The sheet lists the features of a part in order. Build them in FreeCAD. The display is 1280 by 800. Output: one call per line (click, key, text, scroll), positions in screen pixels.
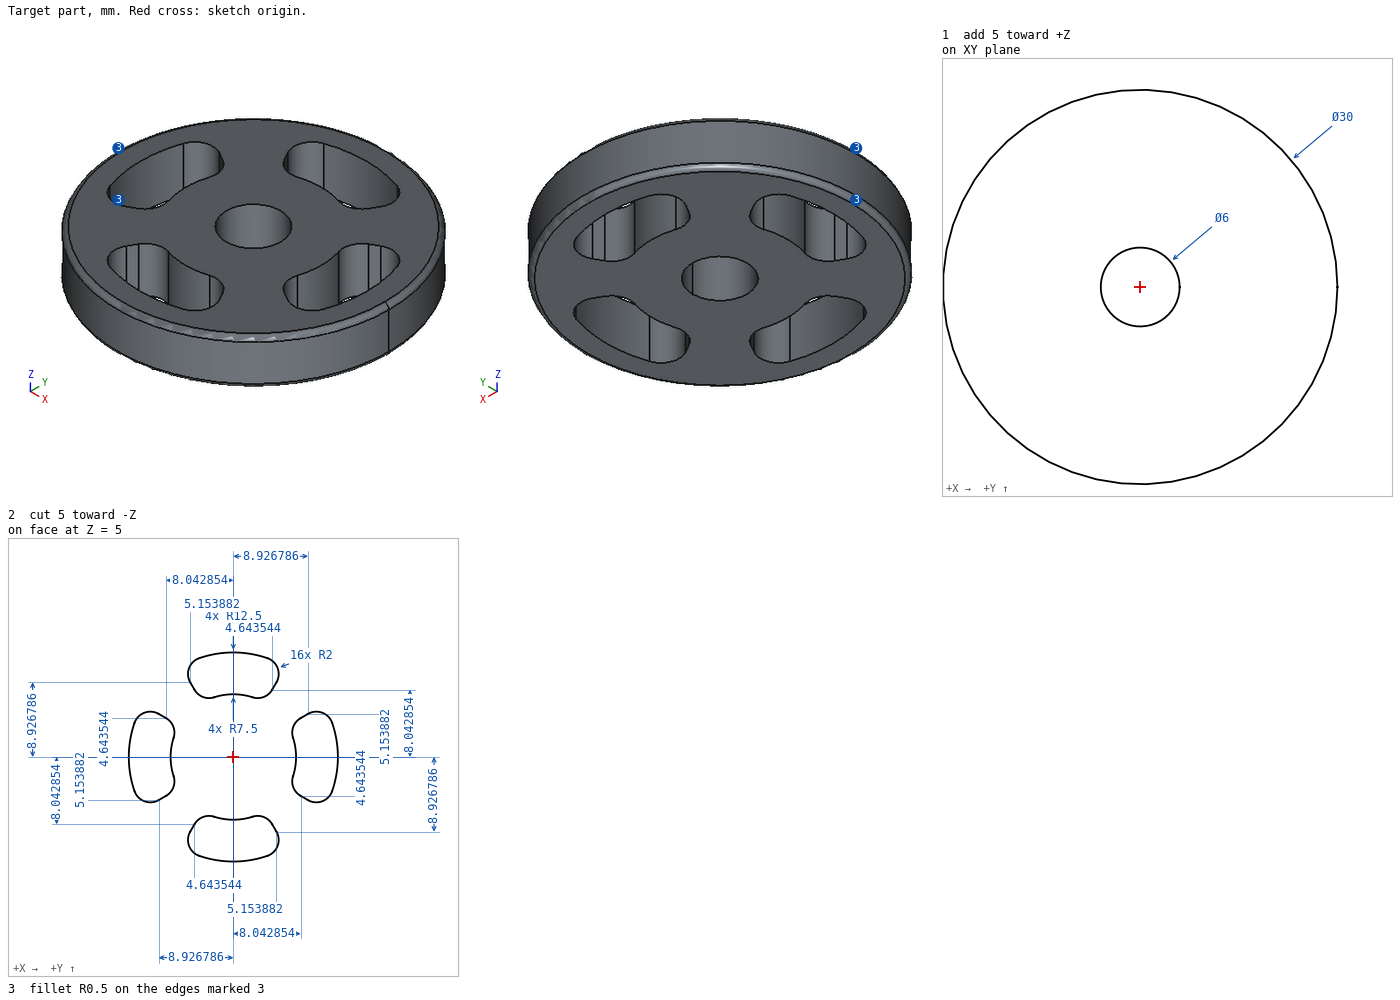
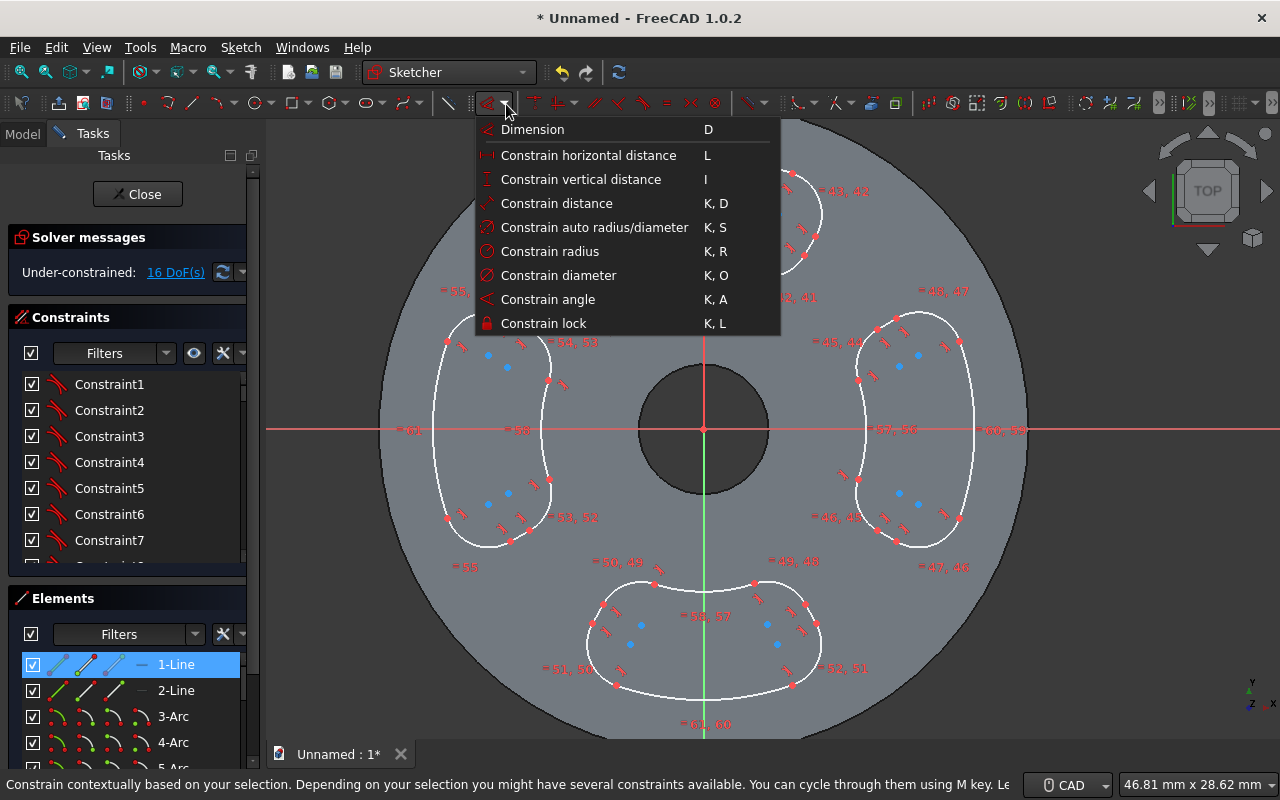
click(628, 155)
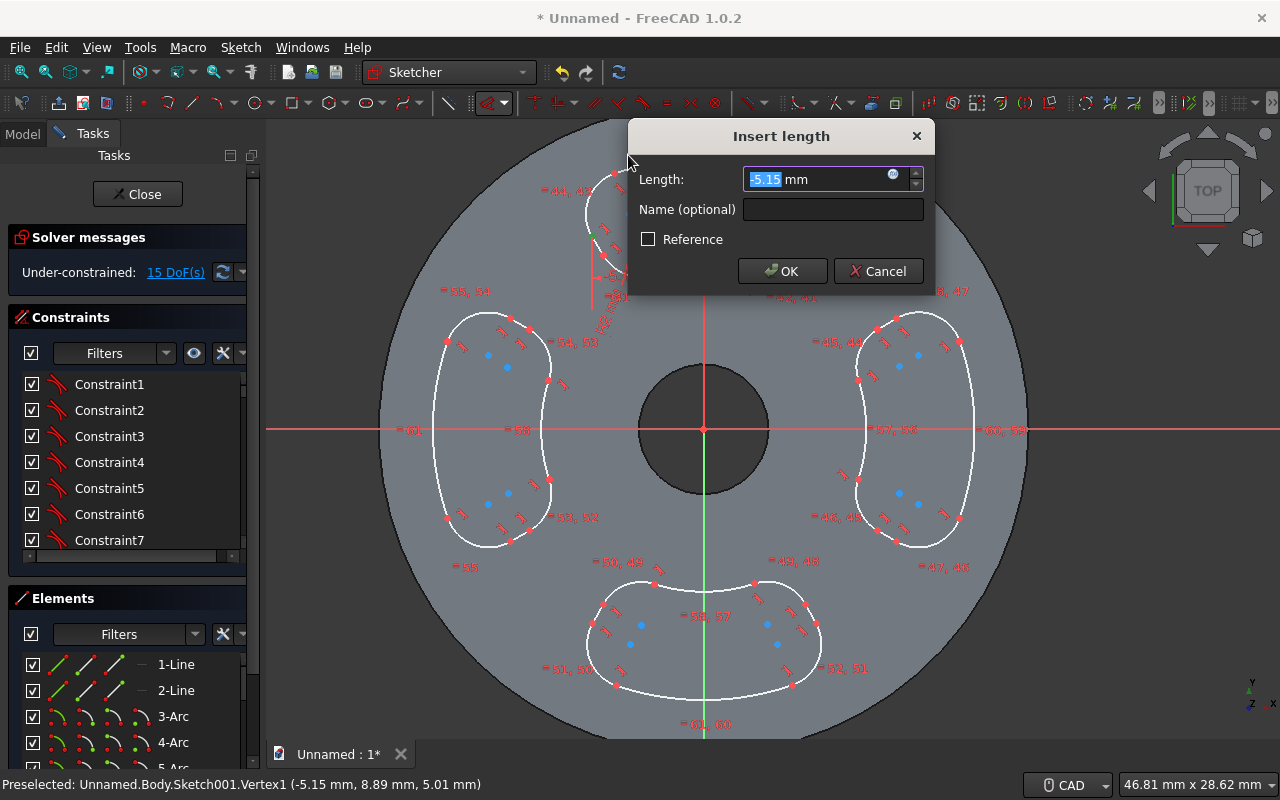
text(-5.153882)
key(Return)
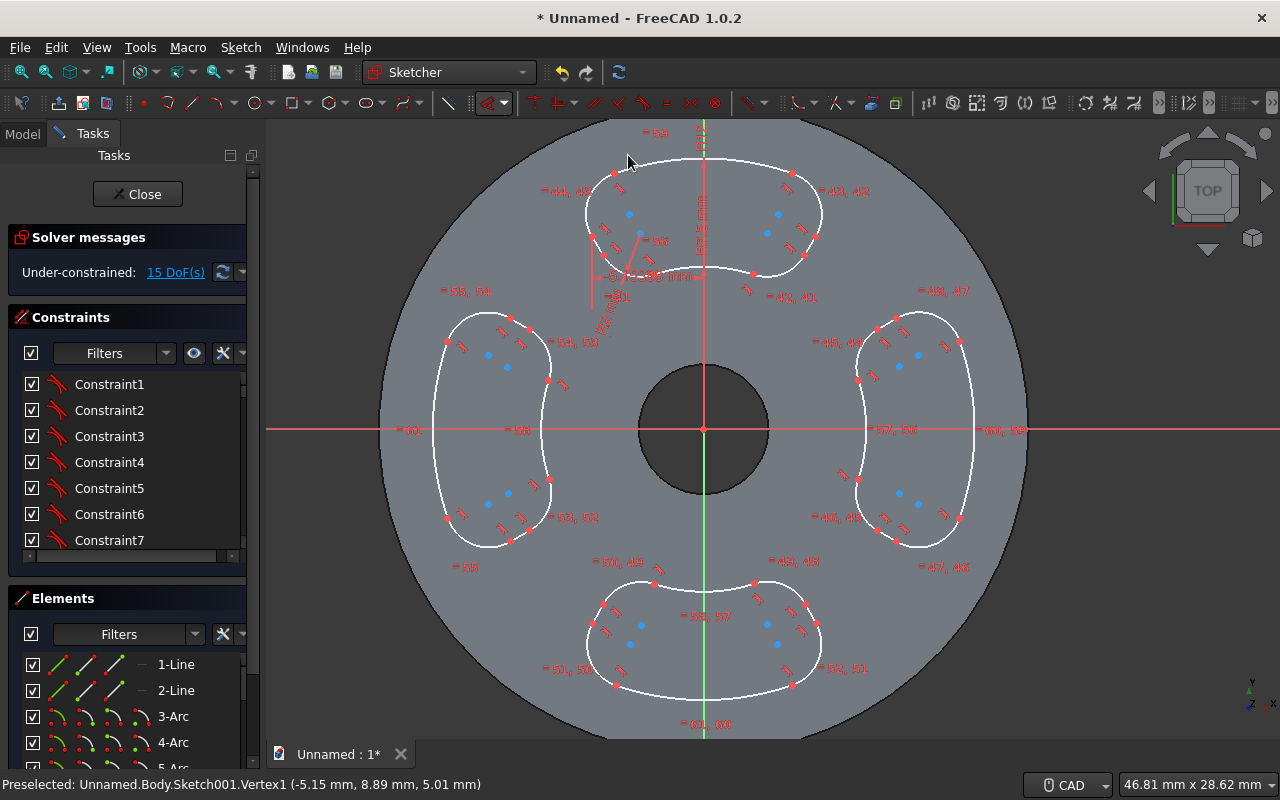
click(592, 237)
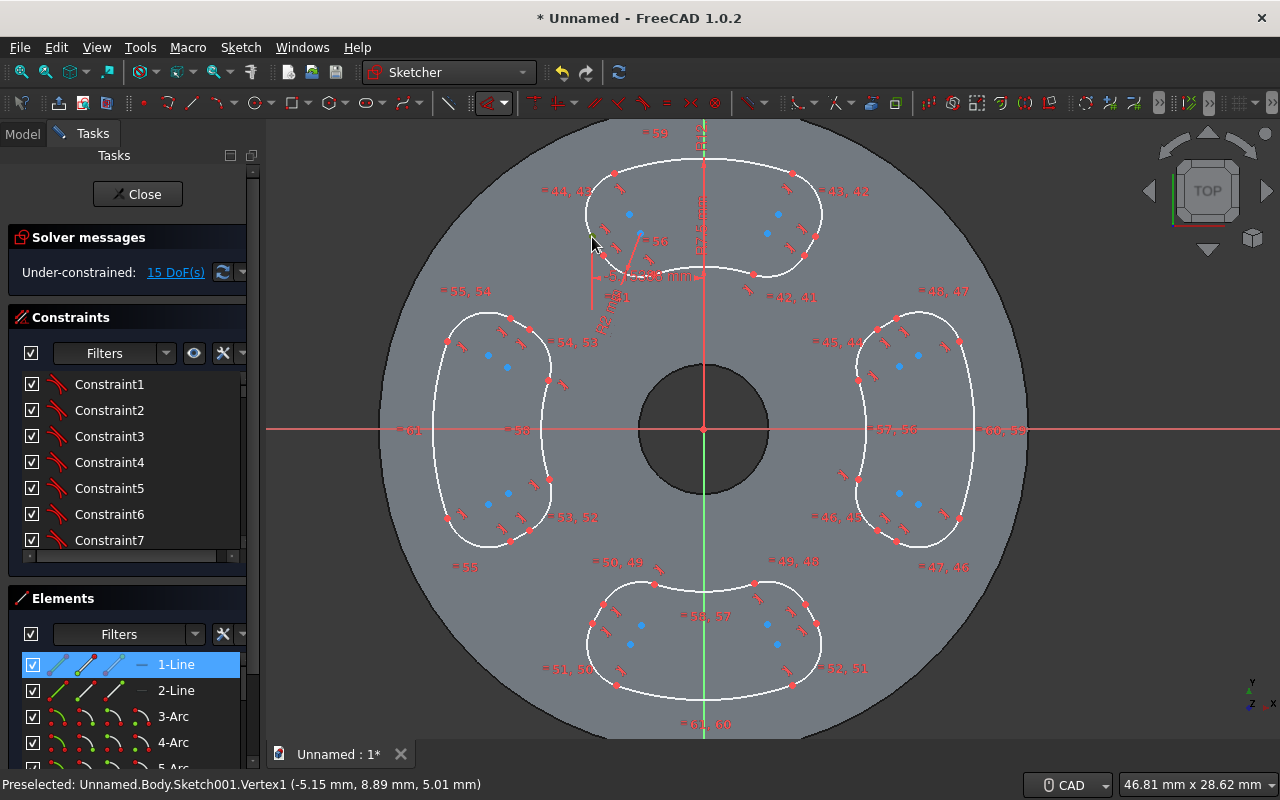
click(506, 104)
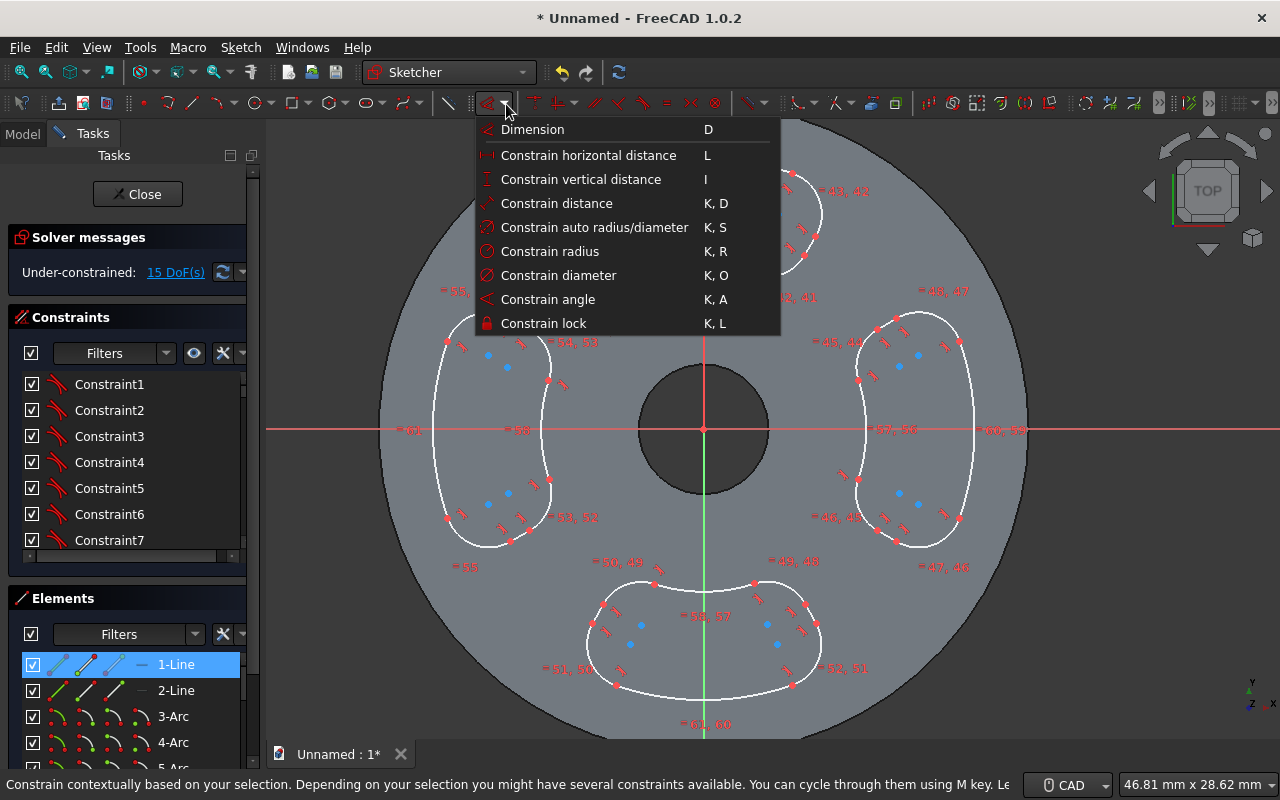
click(628, 179)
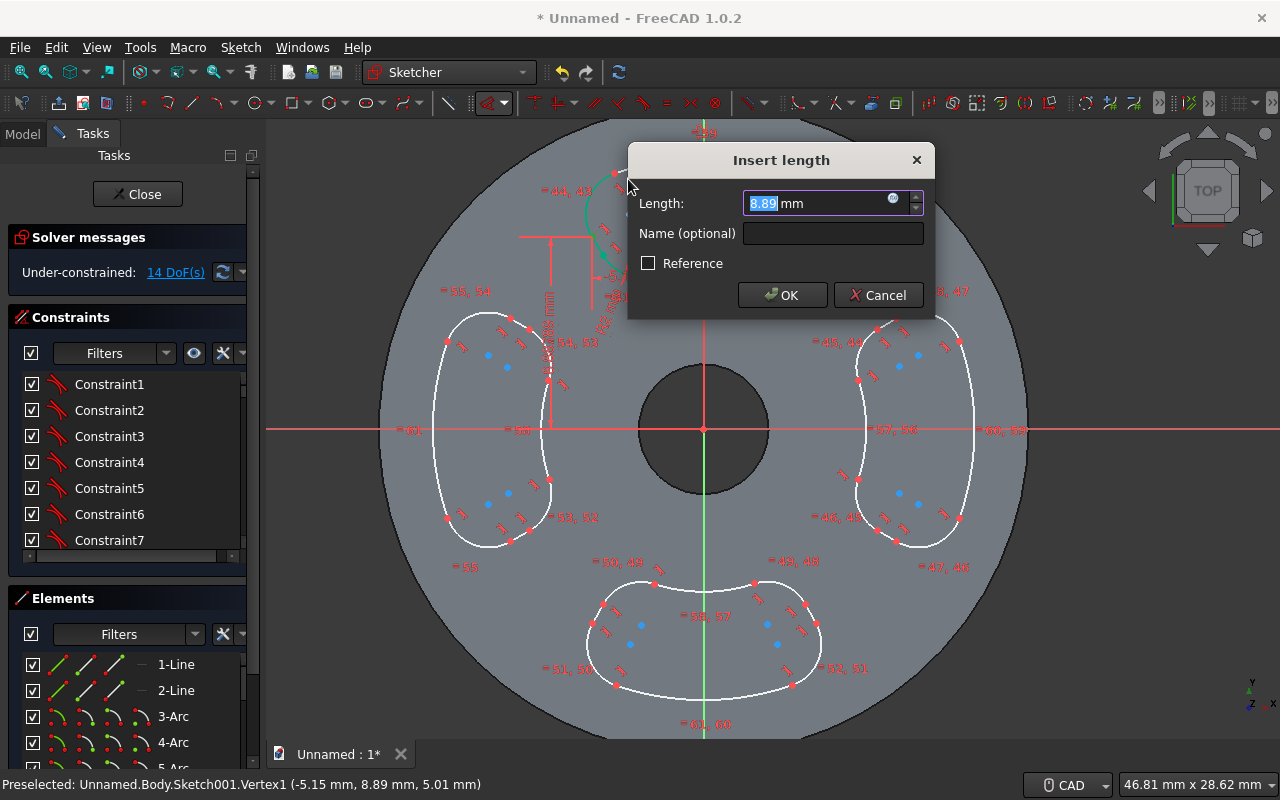
text(8.926786)
key(Return)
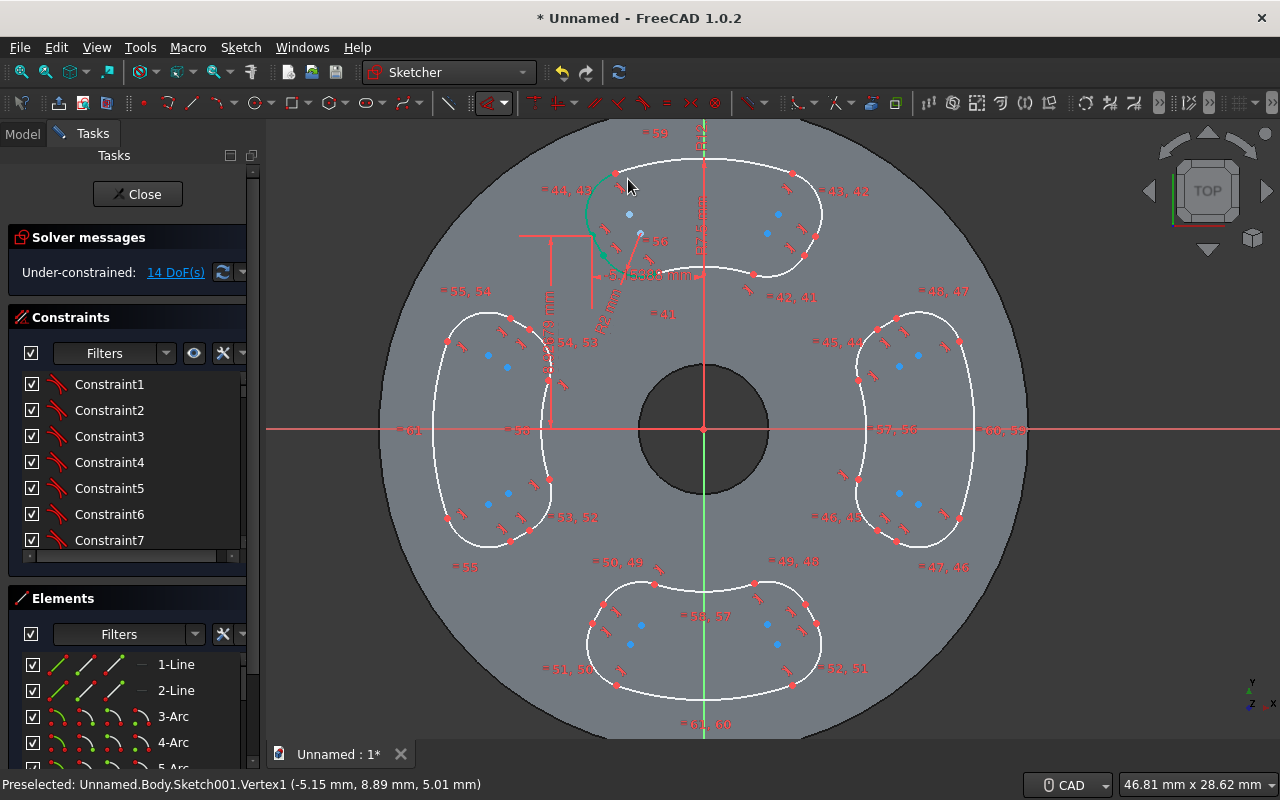
click(804, 256)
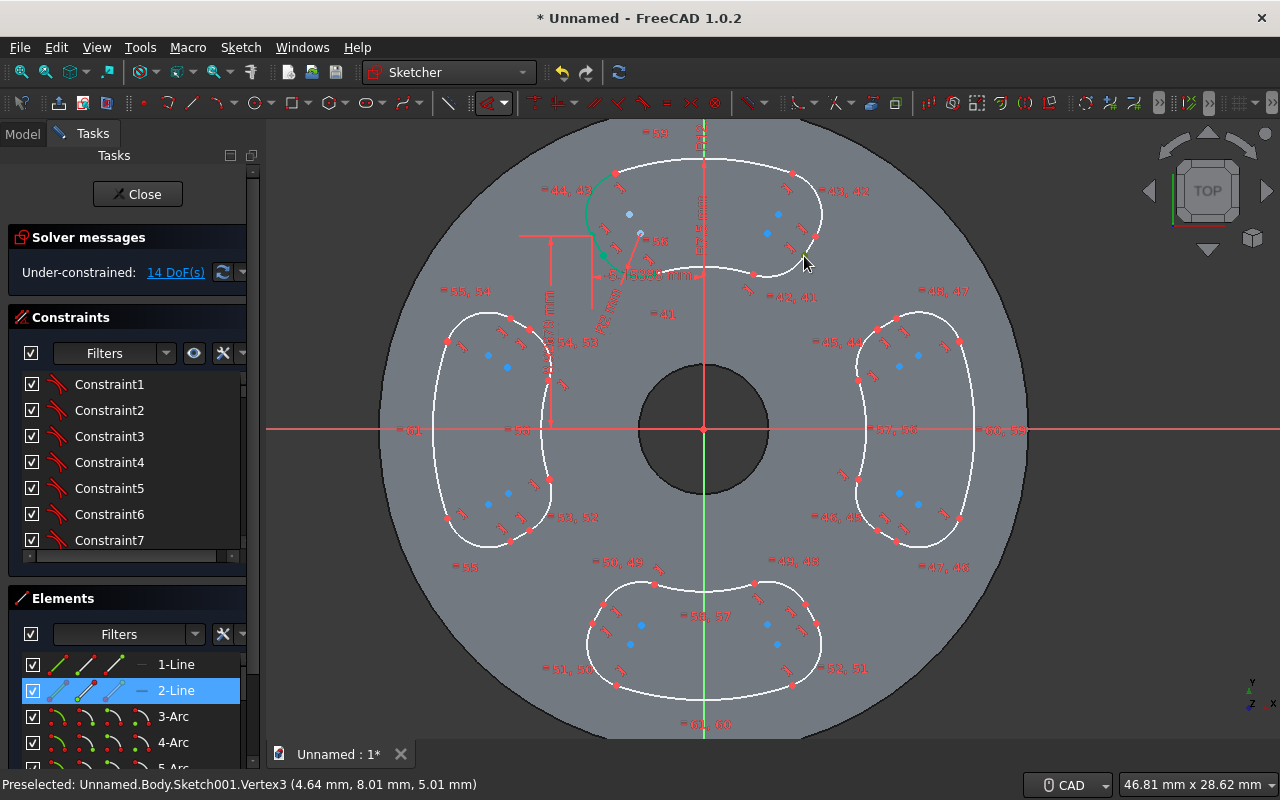
key(l)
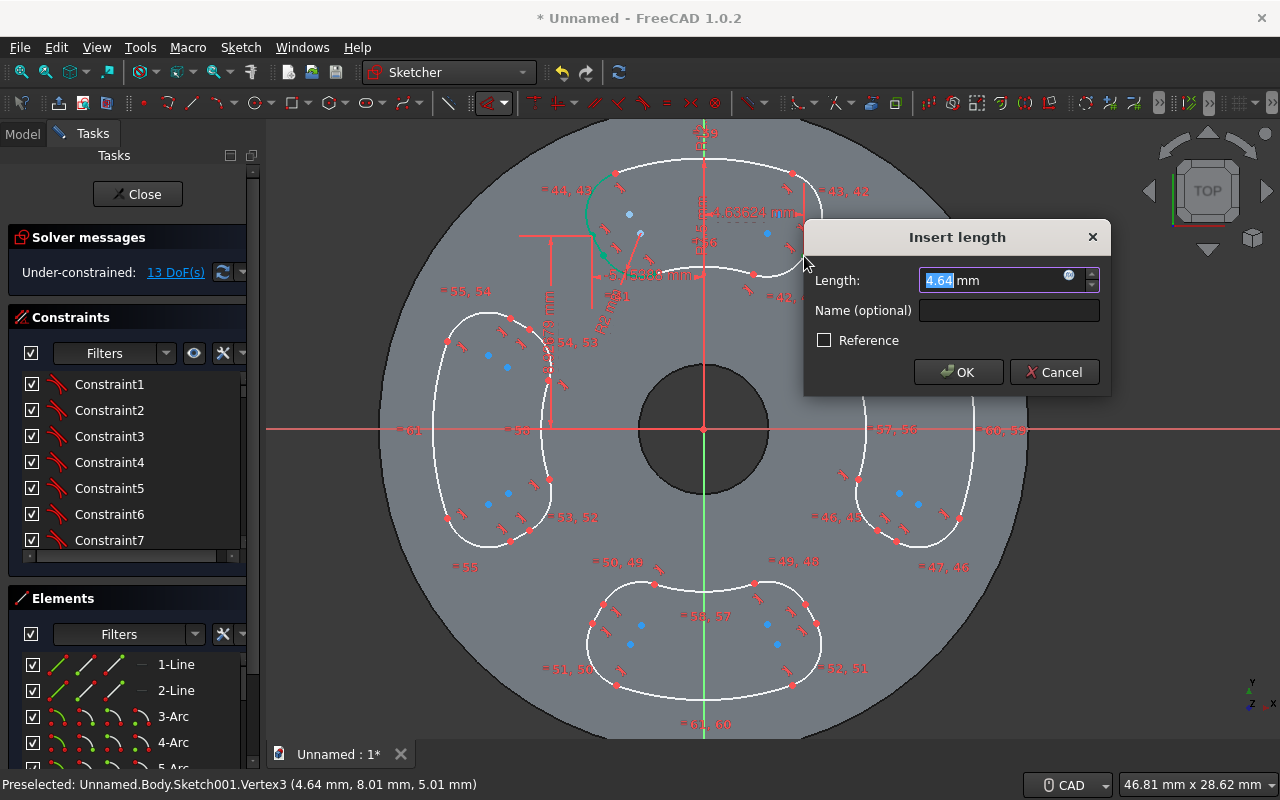
text(4.643544)
key(Return)